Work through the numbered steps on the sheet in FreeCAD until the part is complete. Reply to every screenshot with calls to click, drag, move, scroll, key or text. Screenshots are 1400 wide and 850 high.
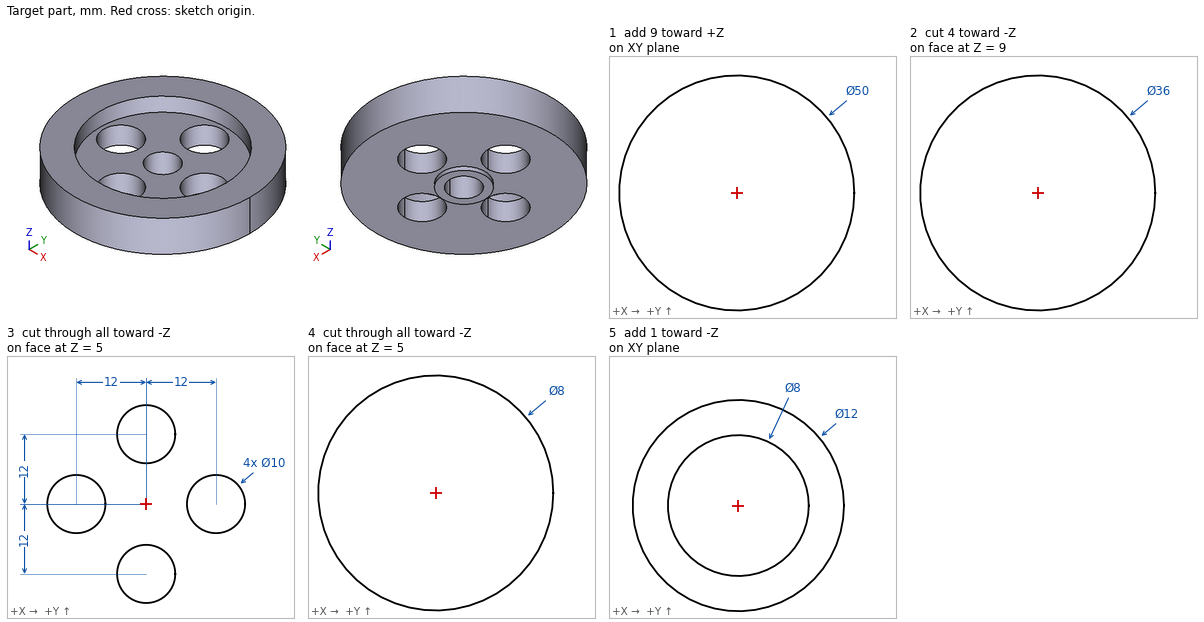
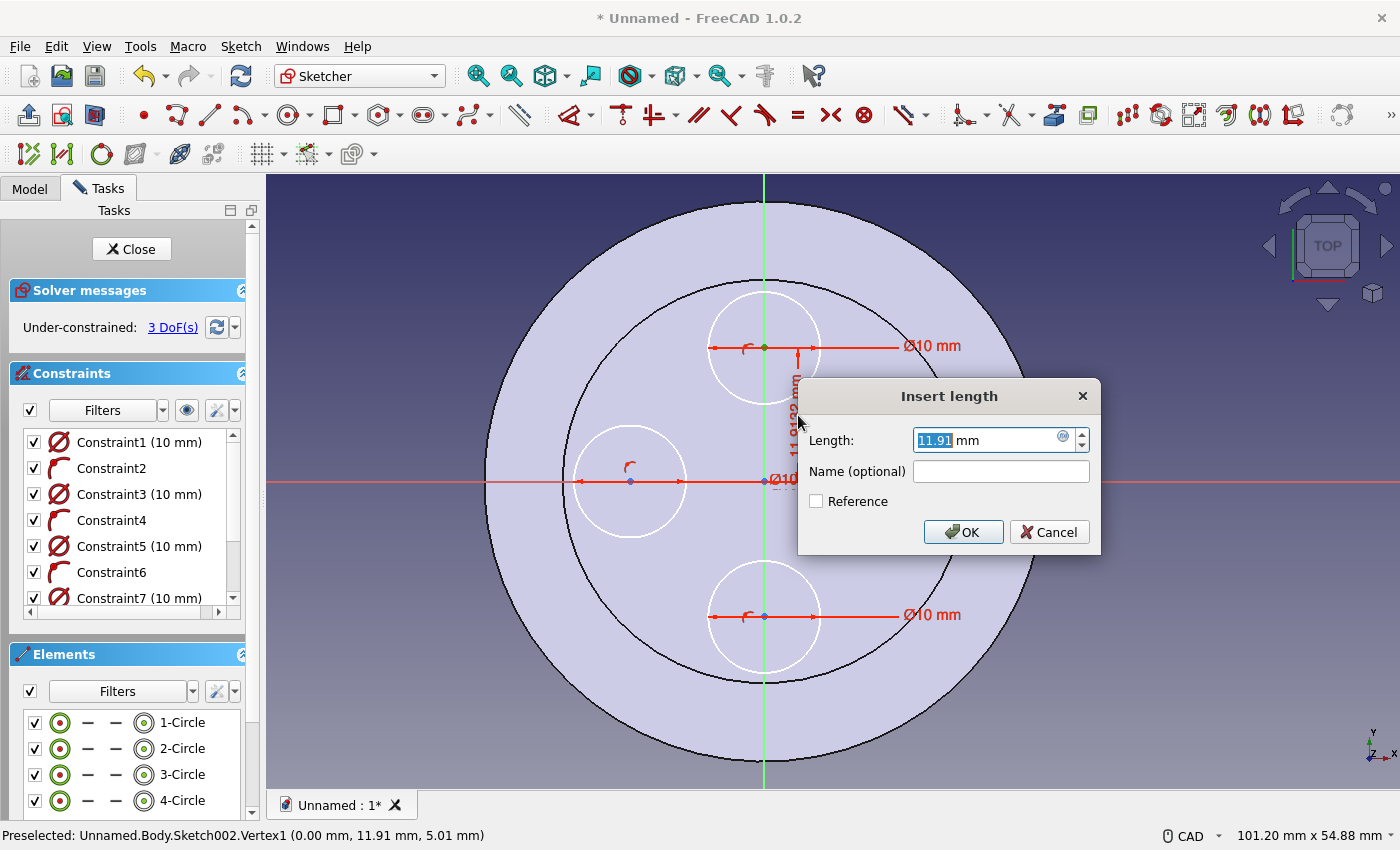
text(12)
key(Return)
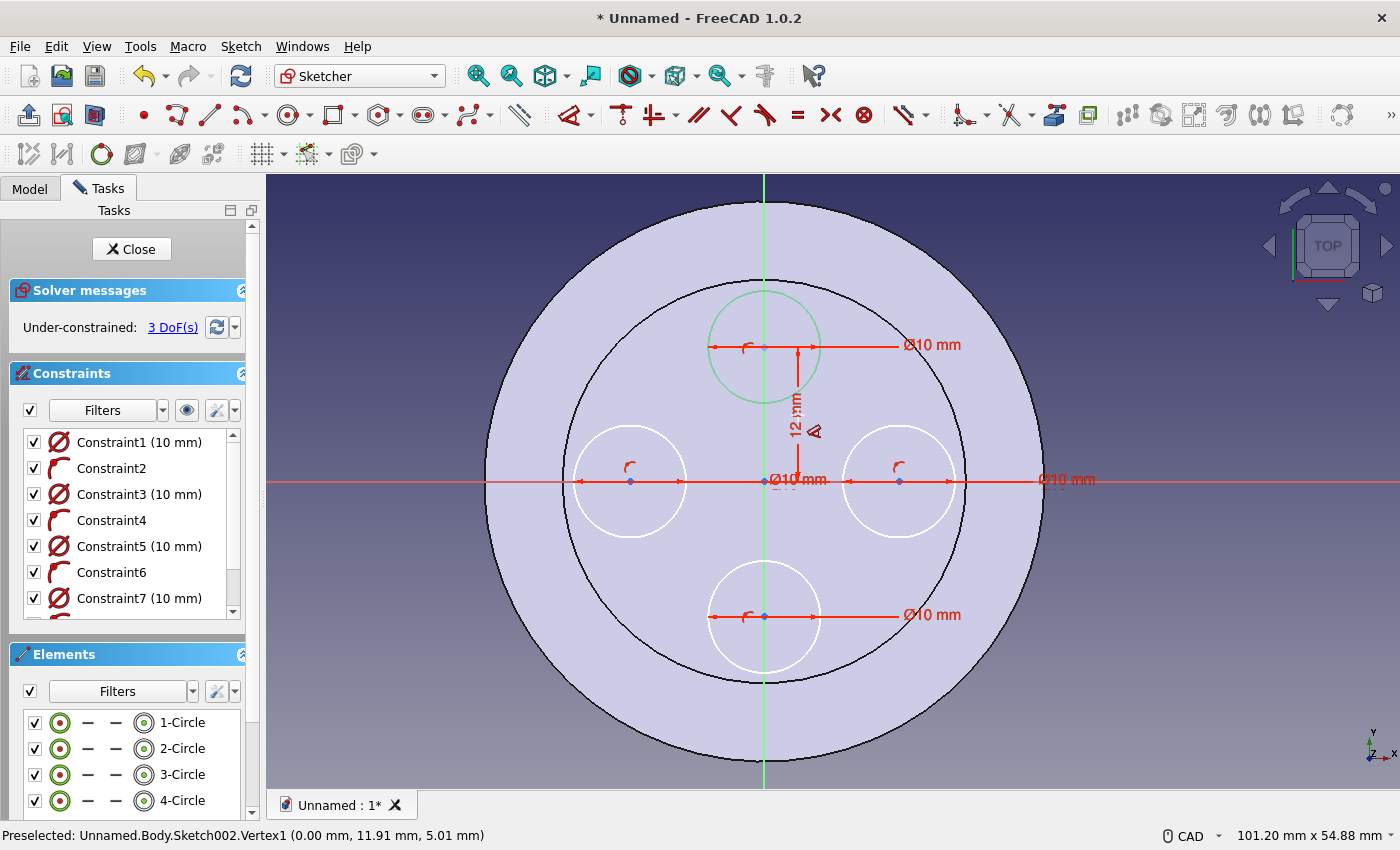
click(899, 482)
click(832, 516)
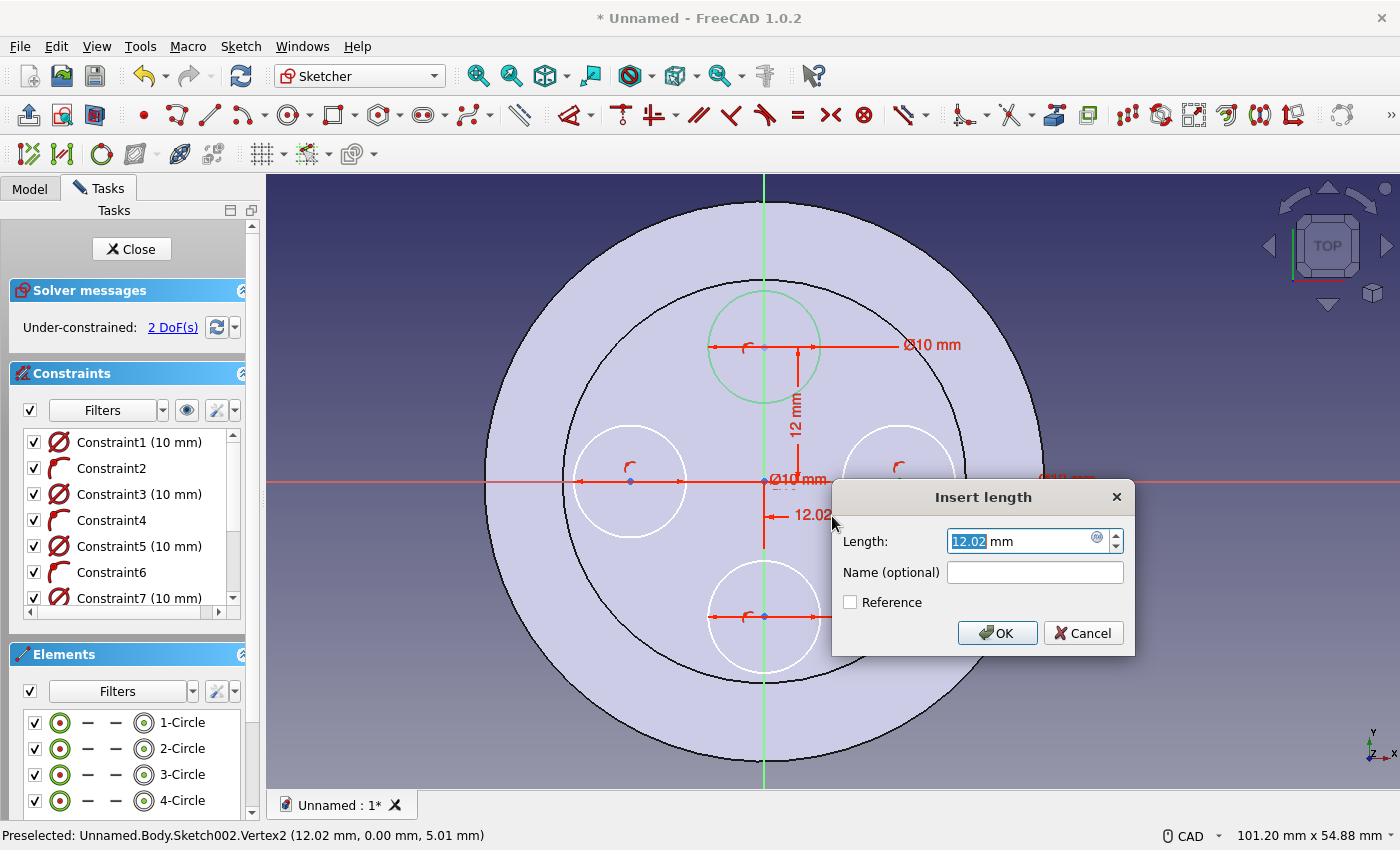
text(12)
key(Return)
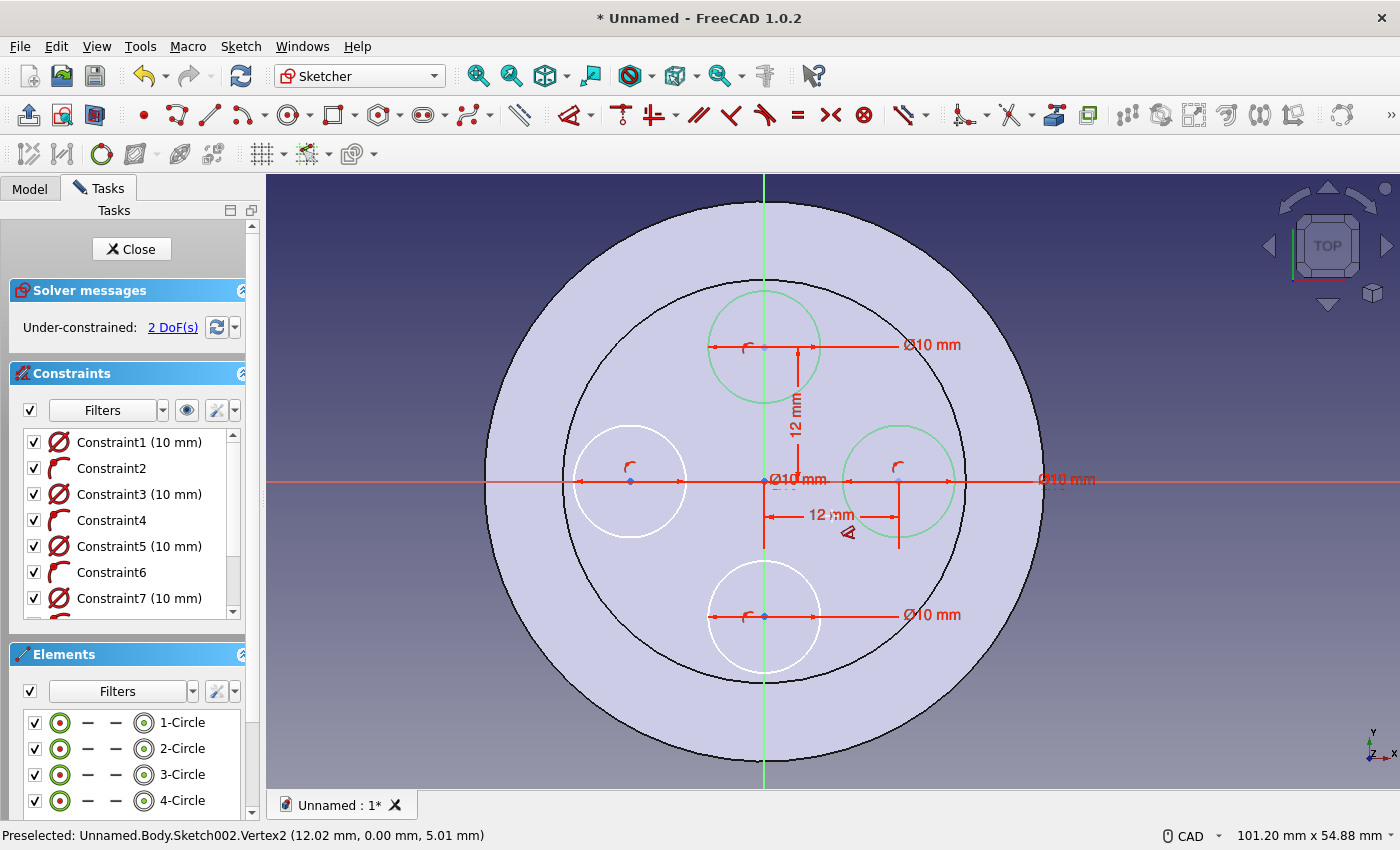
click(764, 617)
click(798, 549)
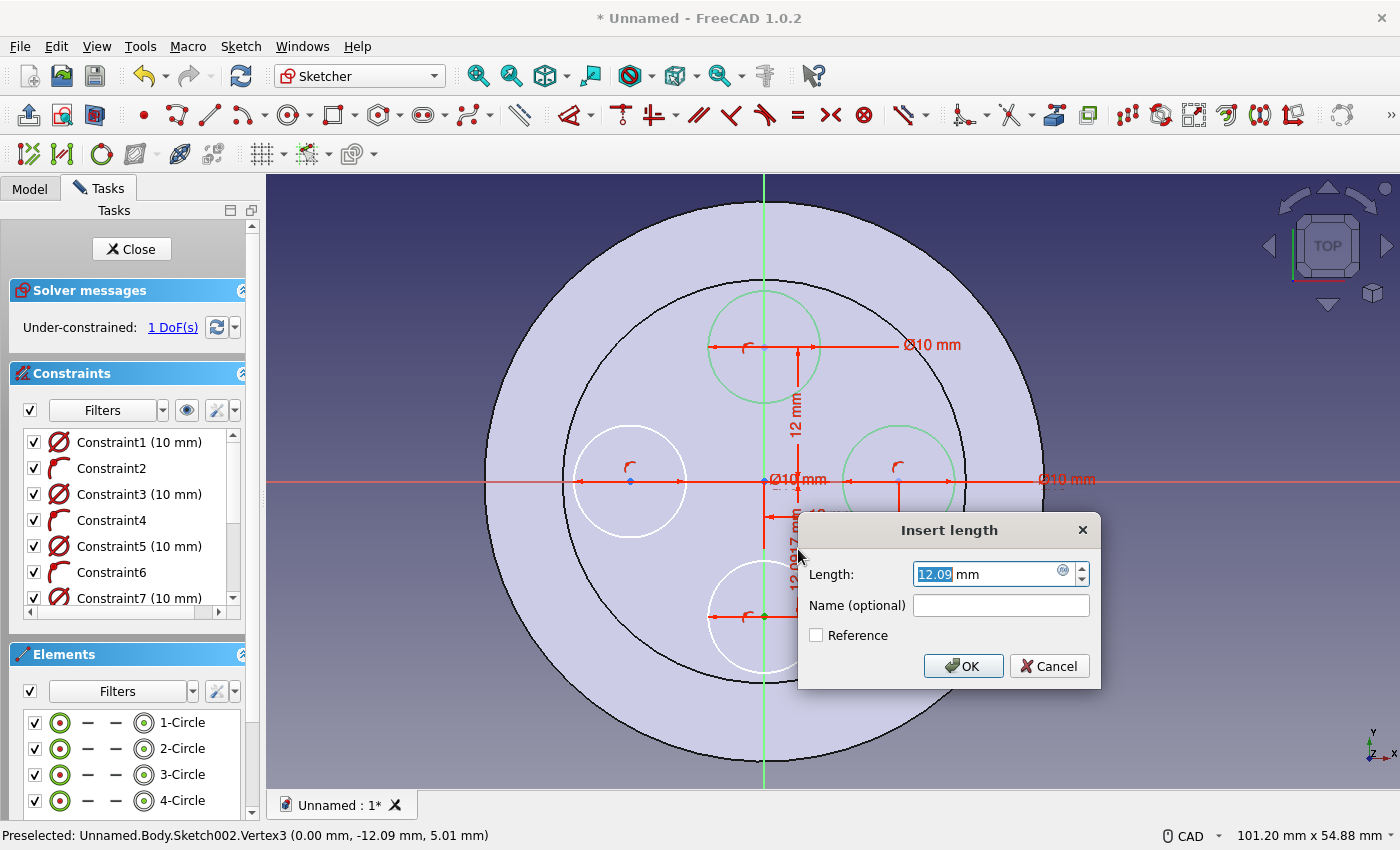
text(12)
key(Return)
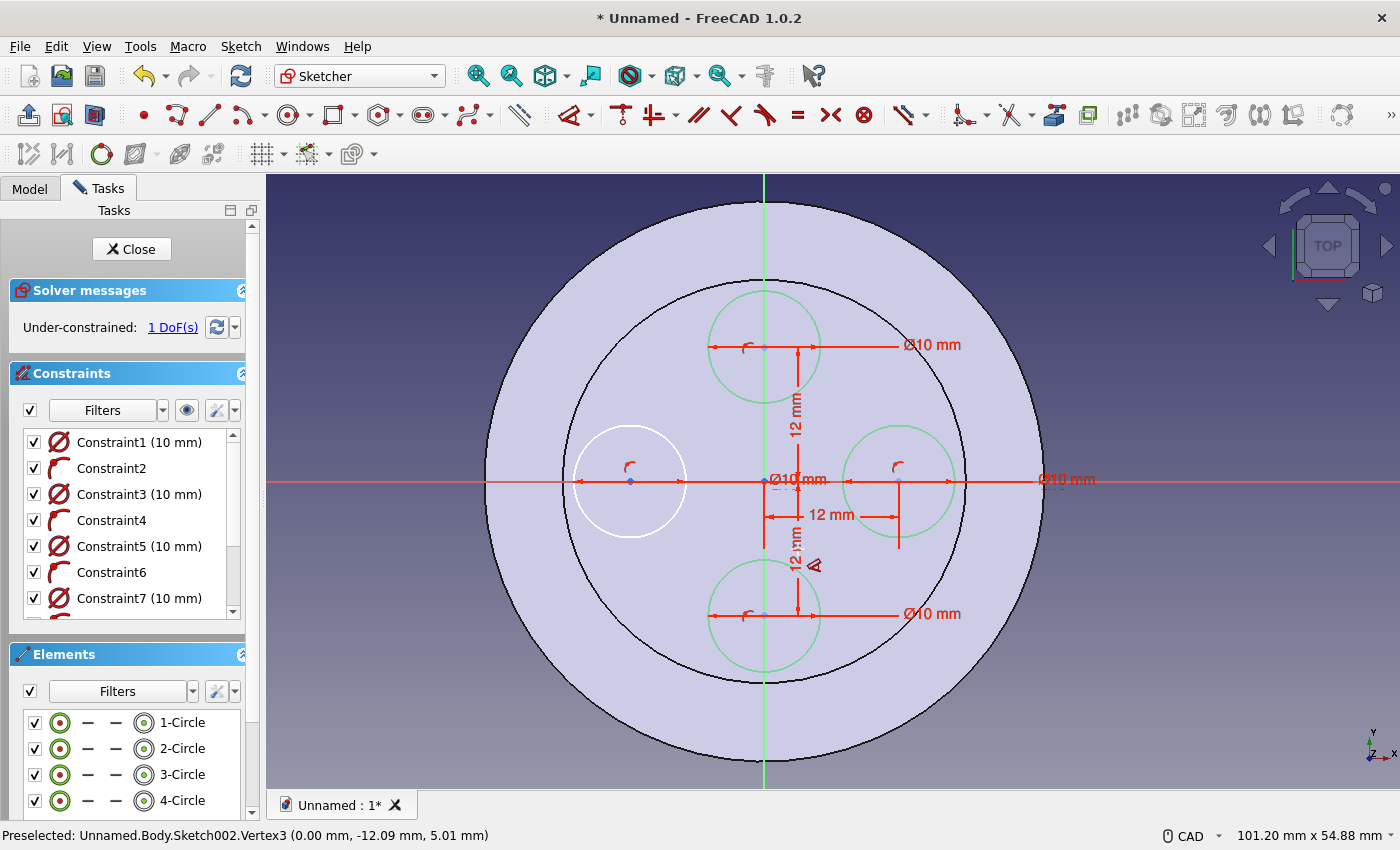
click(630, 482)
click(697, 516)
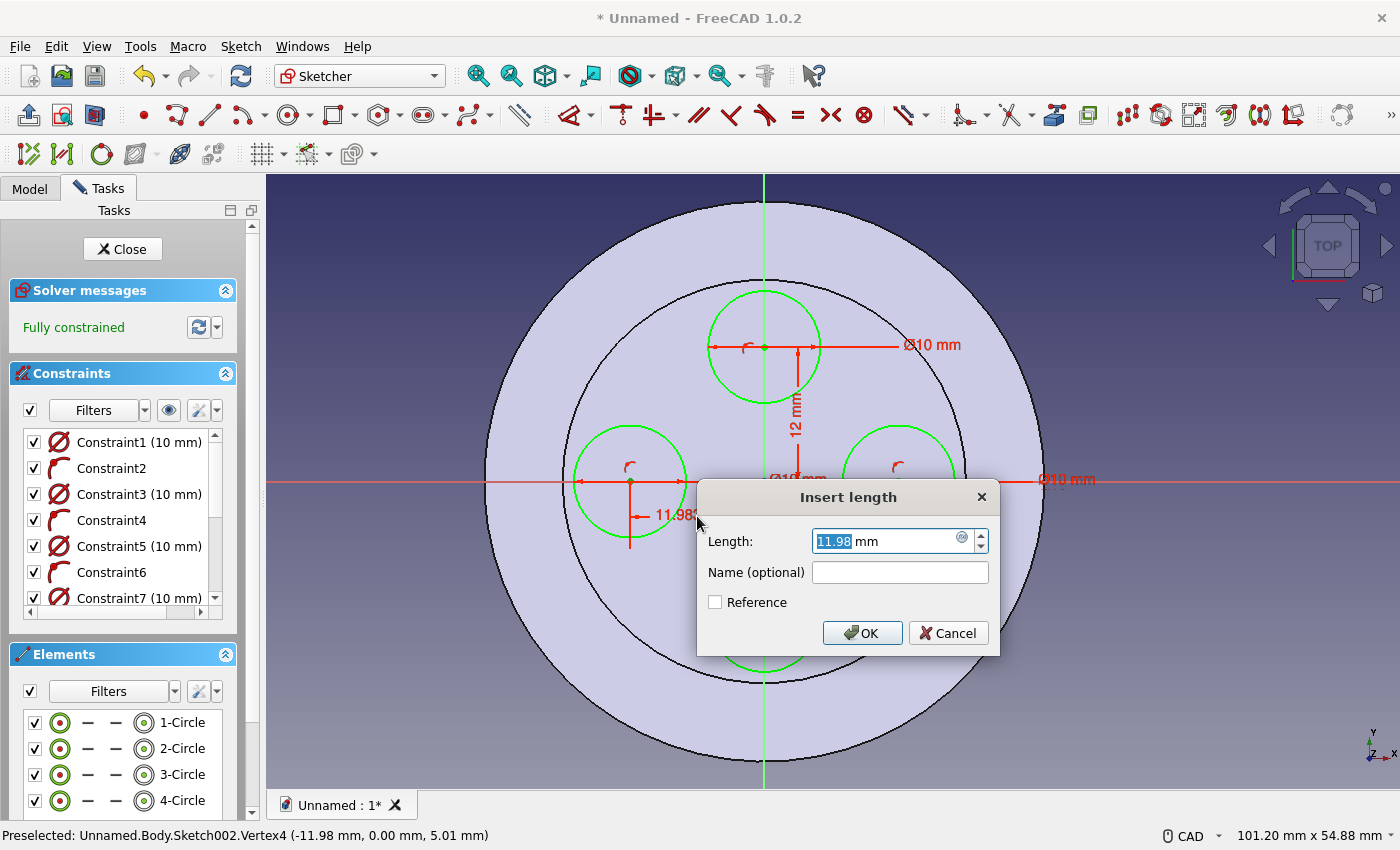
text(12)
key(Return)
key(Escape)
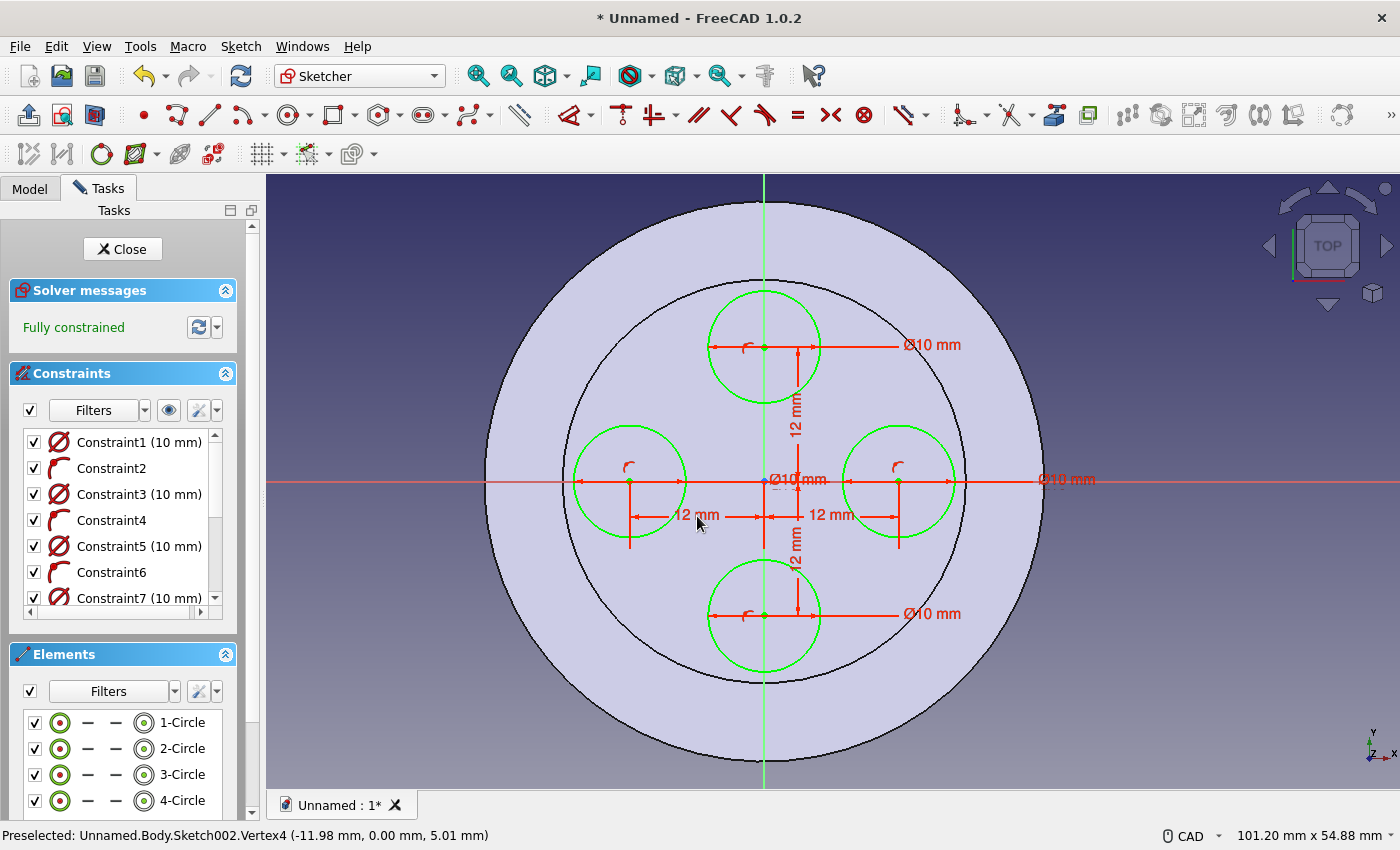
click(123, 249)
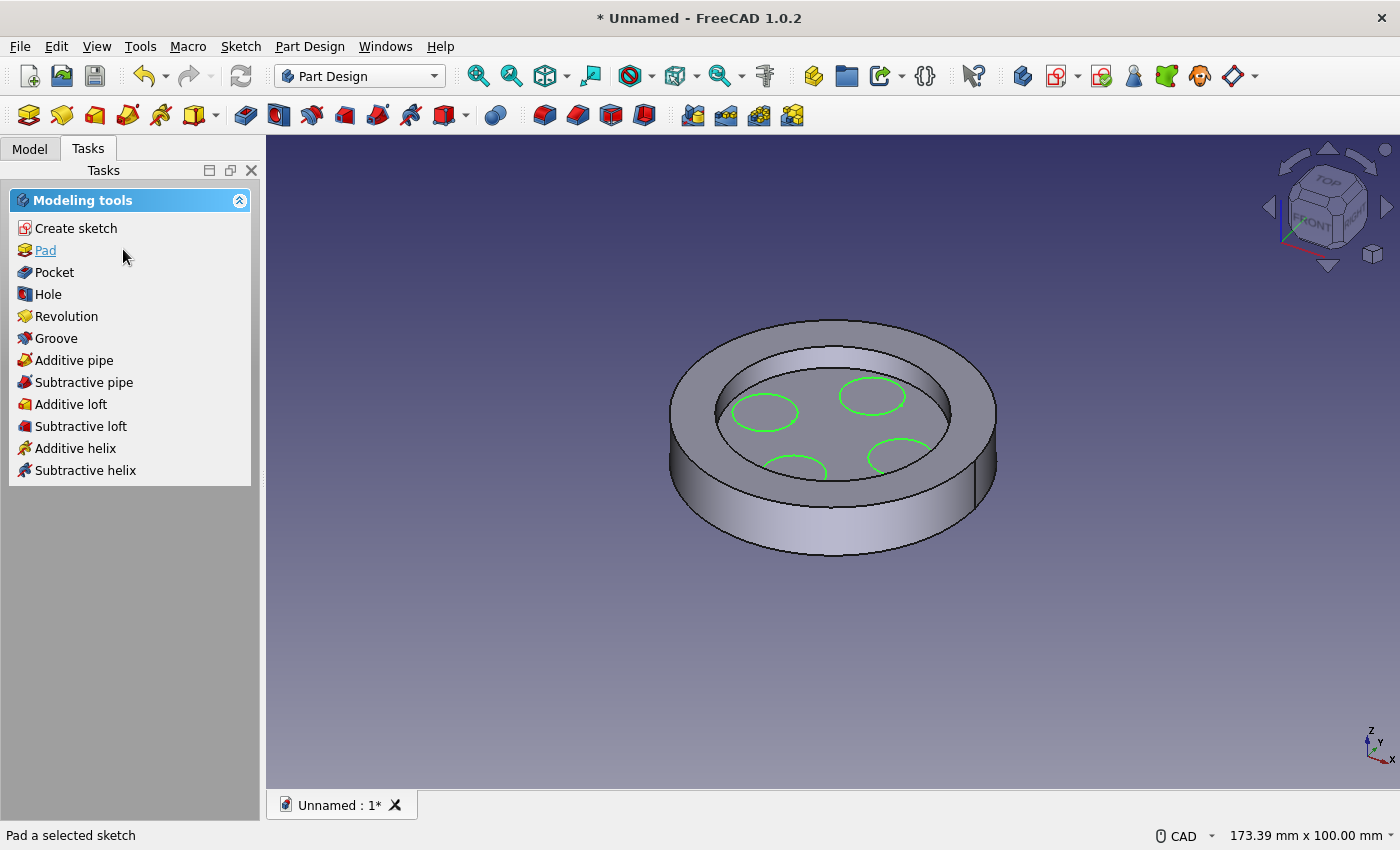
click(246, 116)